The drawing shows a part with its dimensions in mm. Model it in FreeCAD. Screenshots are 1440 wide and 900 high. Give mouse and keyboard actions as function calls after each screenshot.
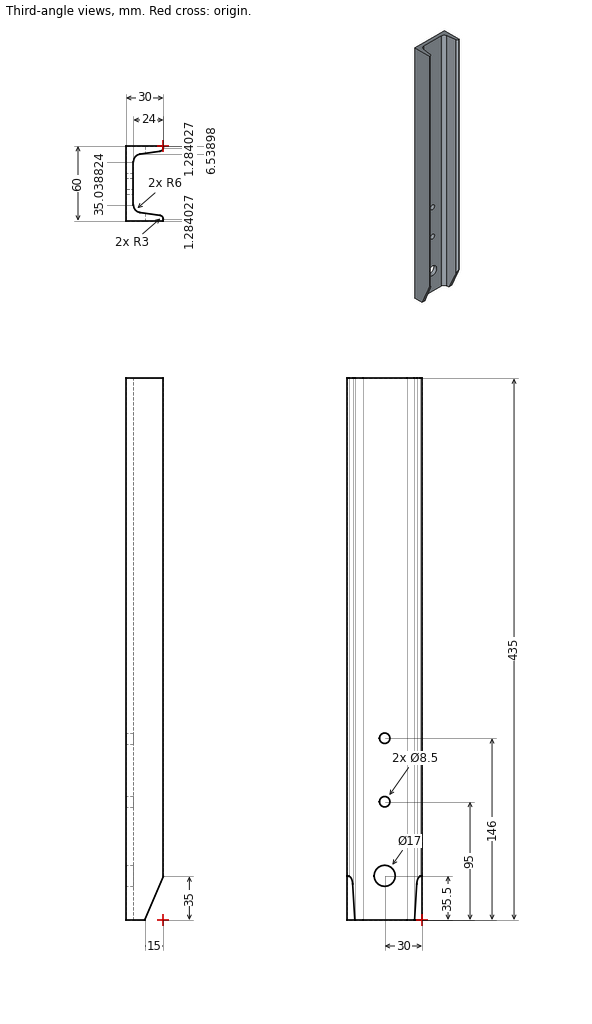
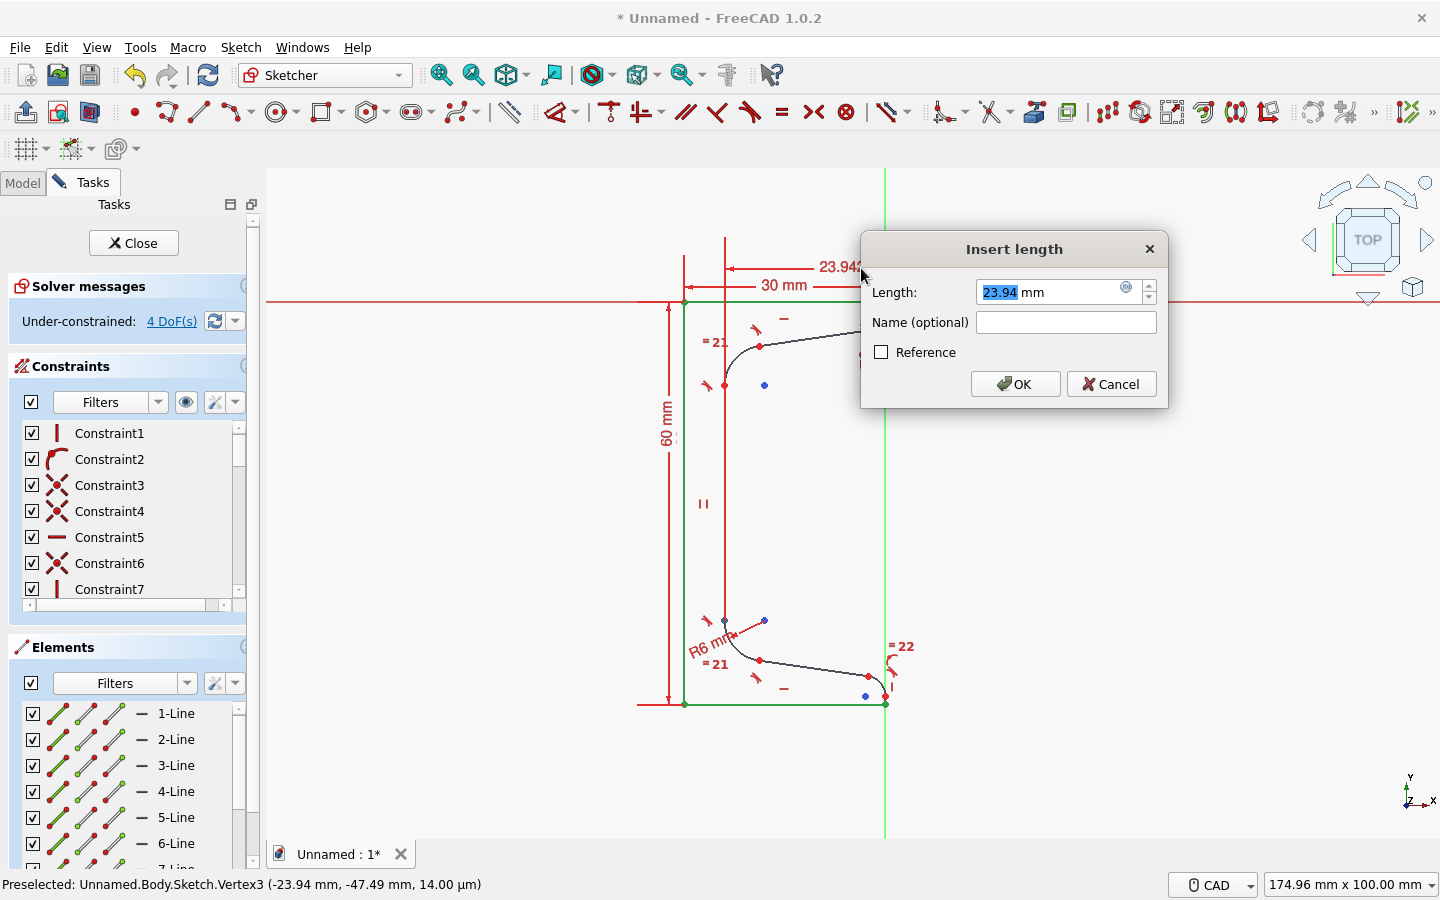
text(24)
key(Return)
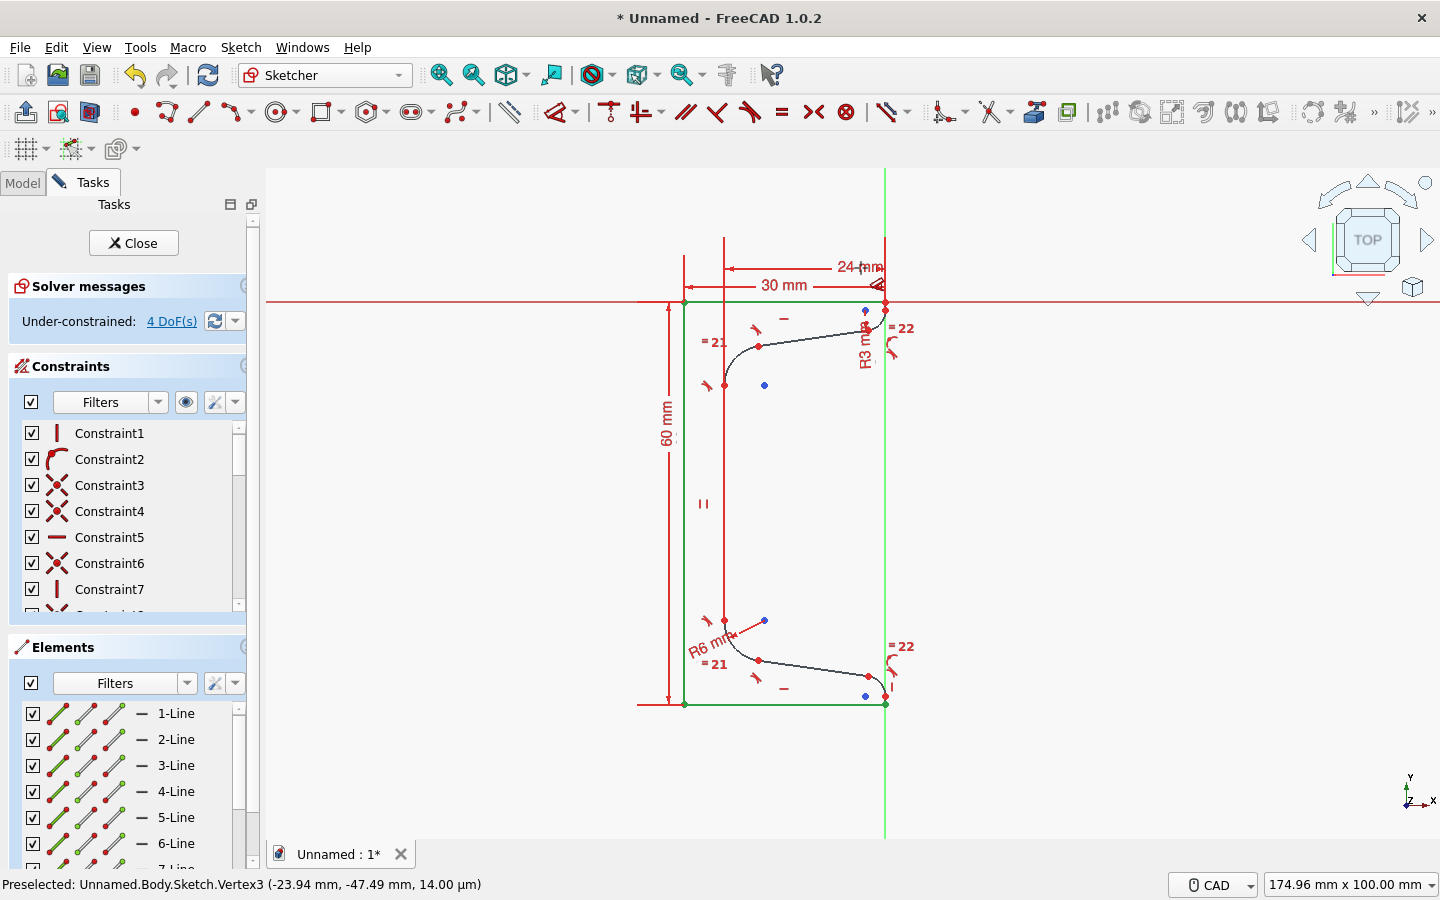
scroll(885, 306, up, 8)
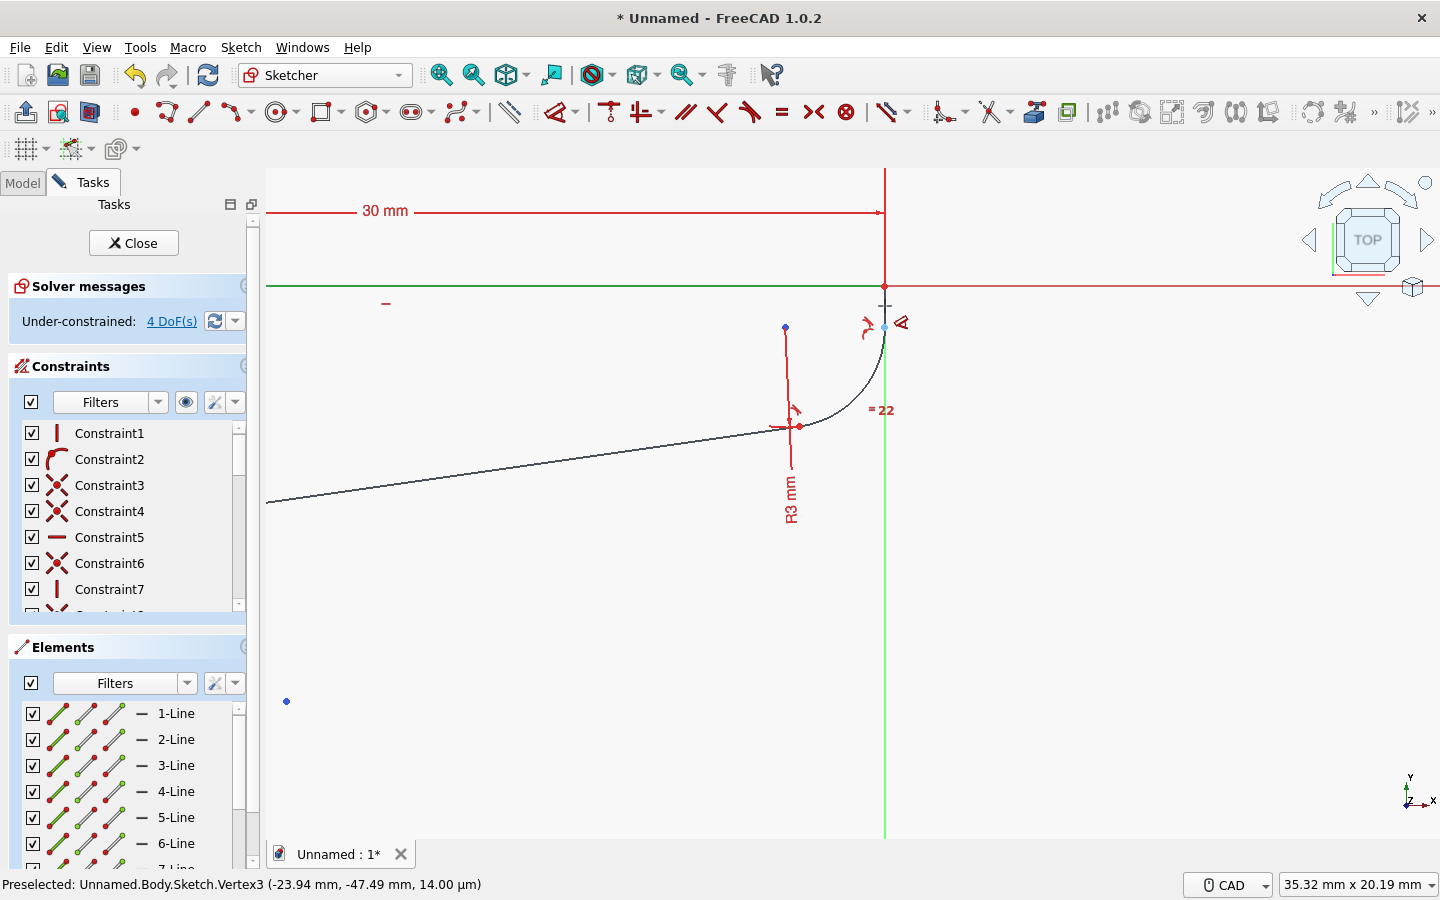
click(885, 307)
click(919, 307)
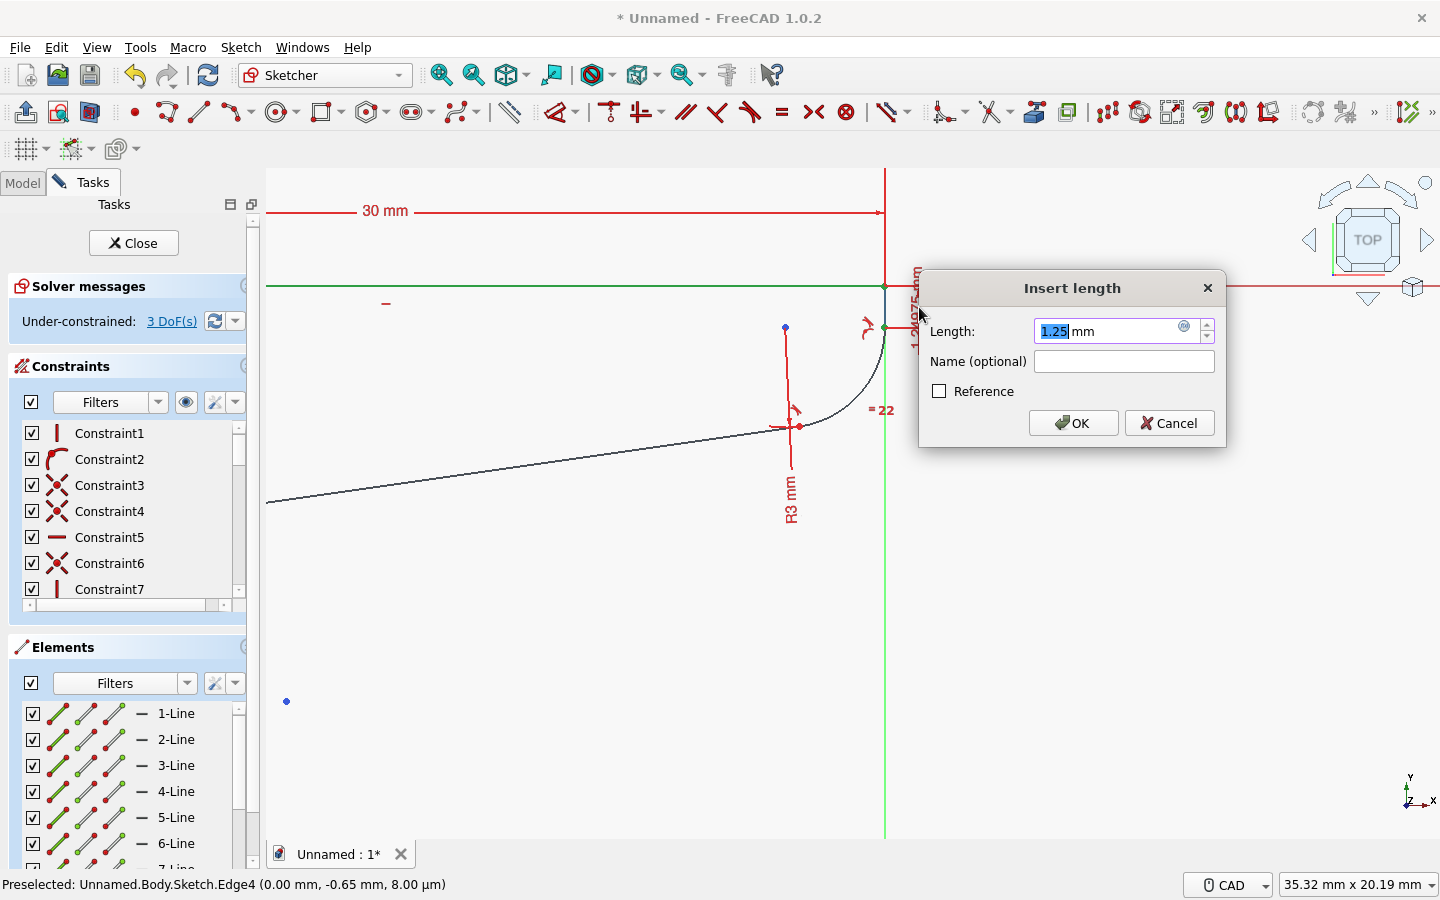
text(1.284027)
key(Return)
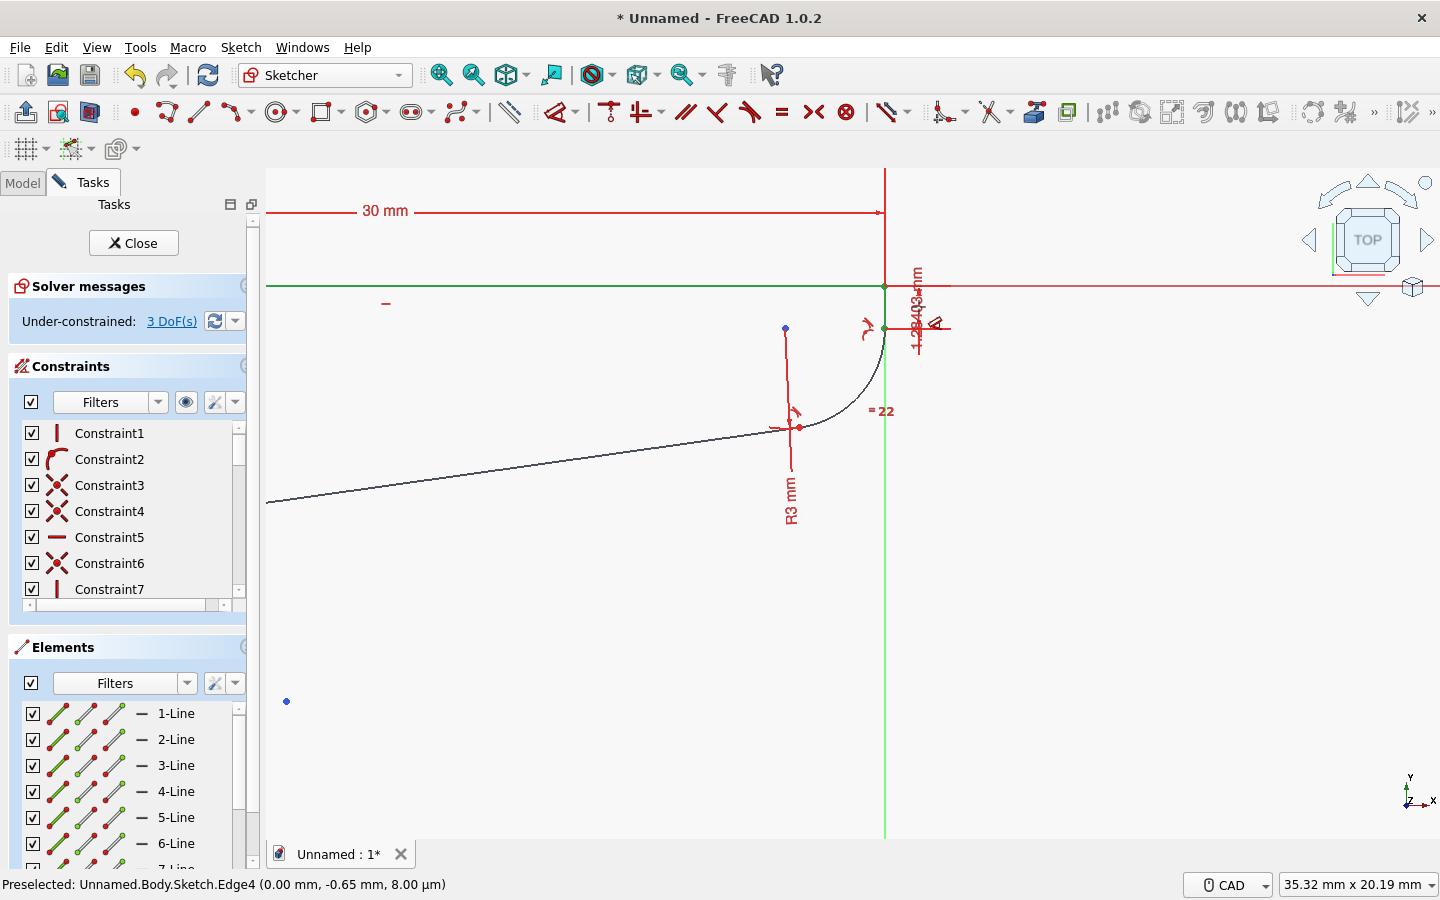
scroll(885, 306, down, 8)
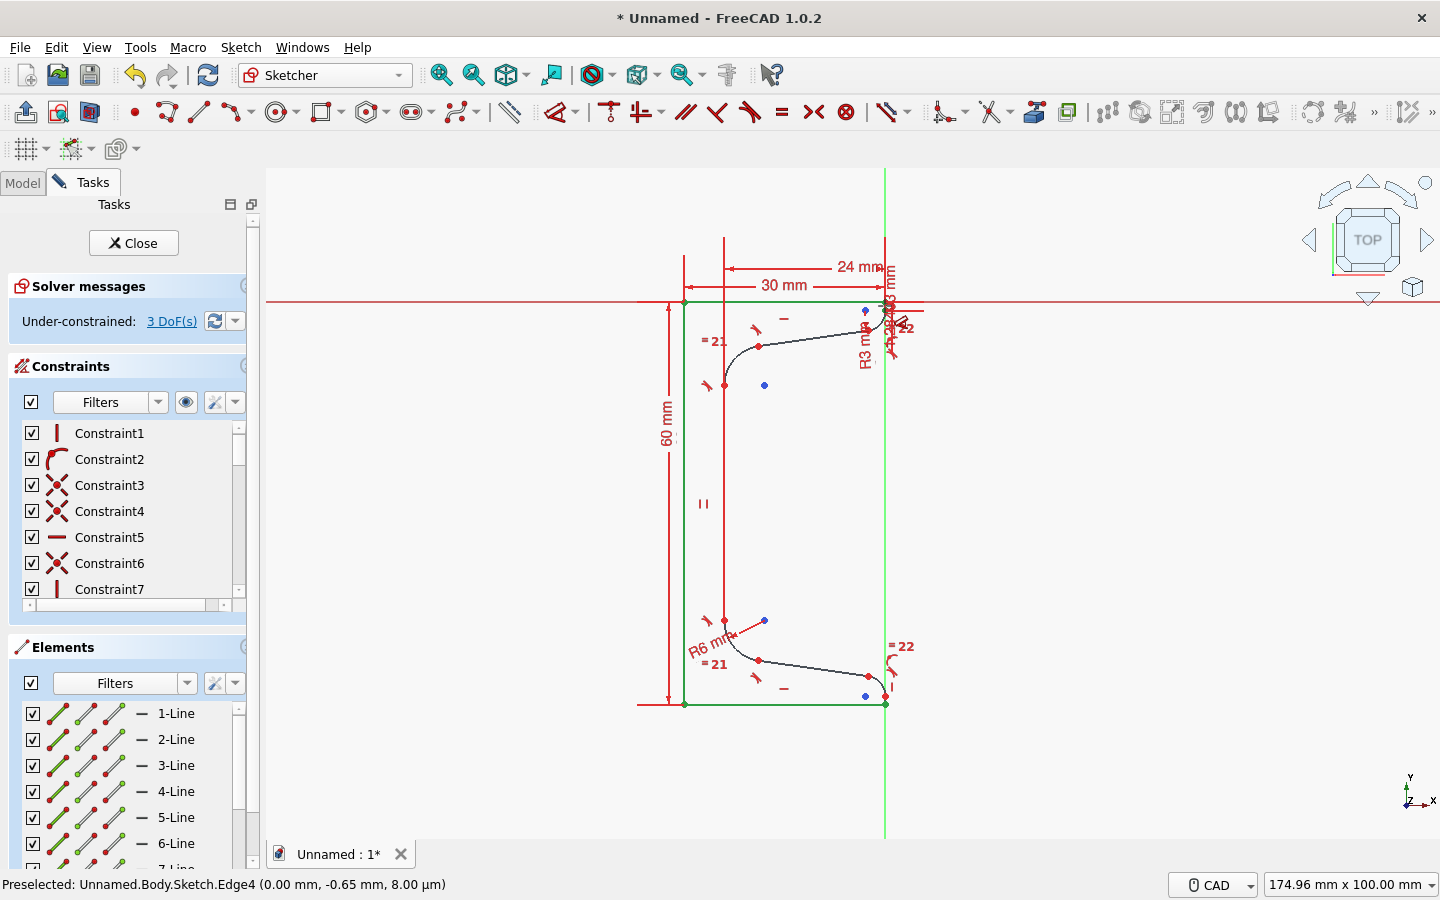
scroll(885, 702, up, 9)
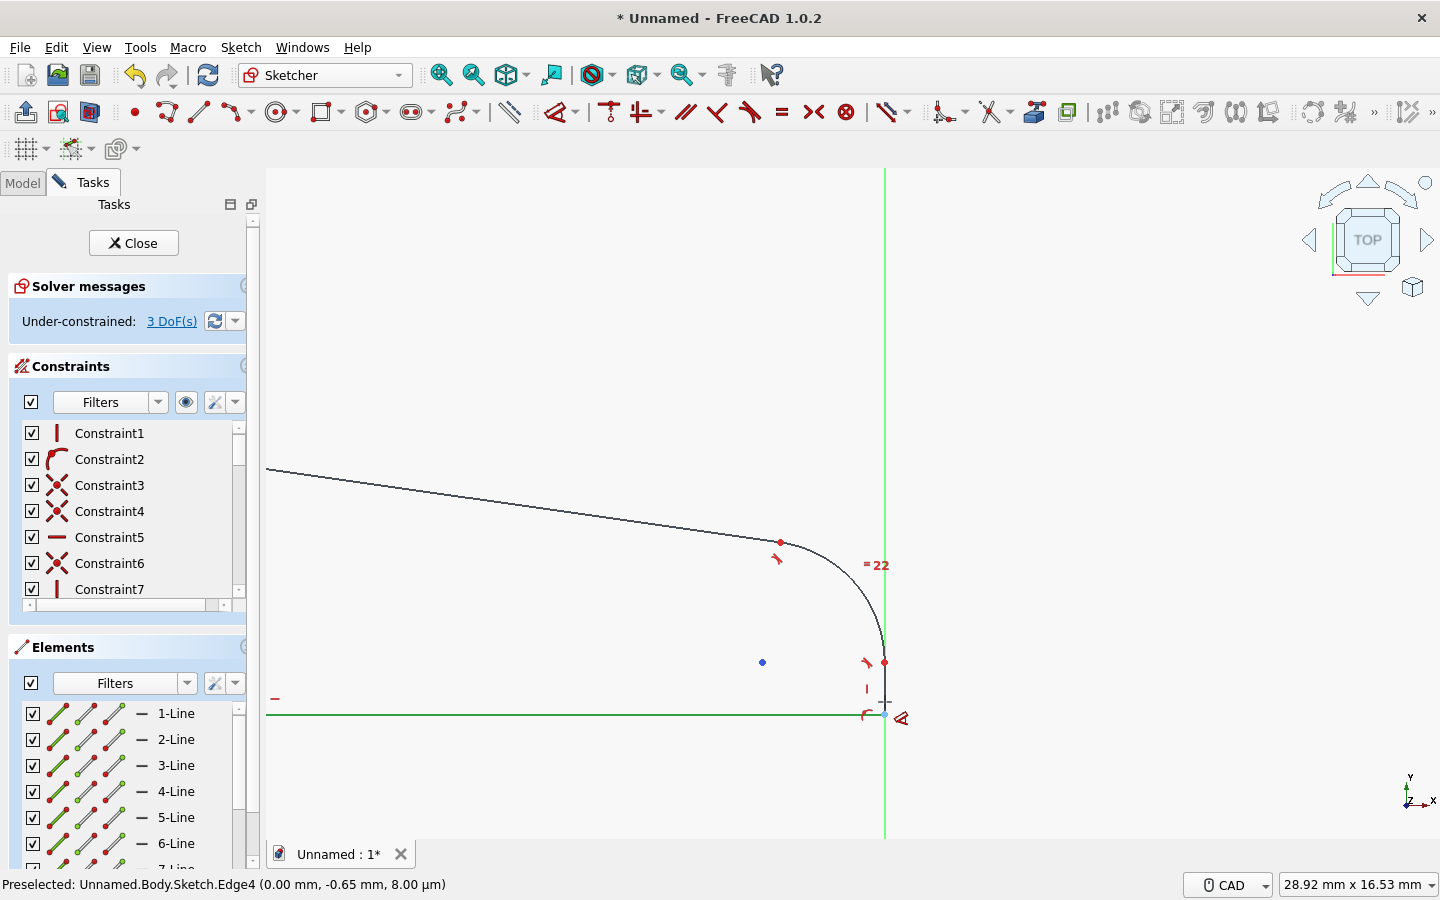
click(885, 699)
click(919, 689)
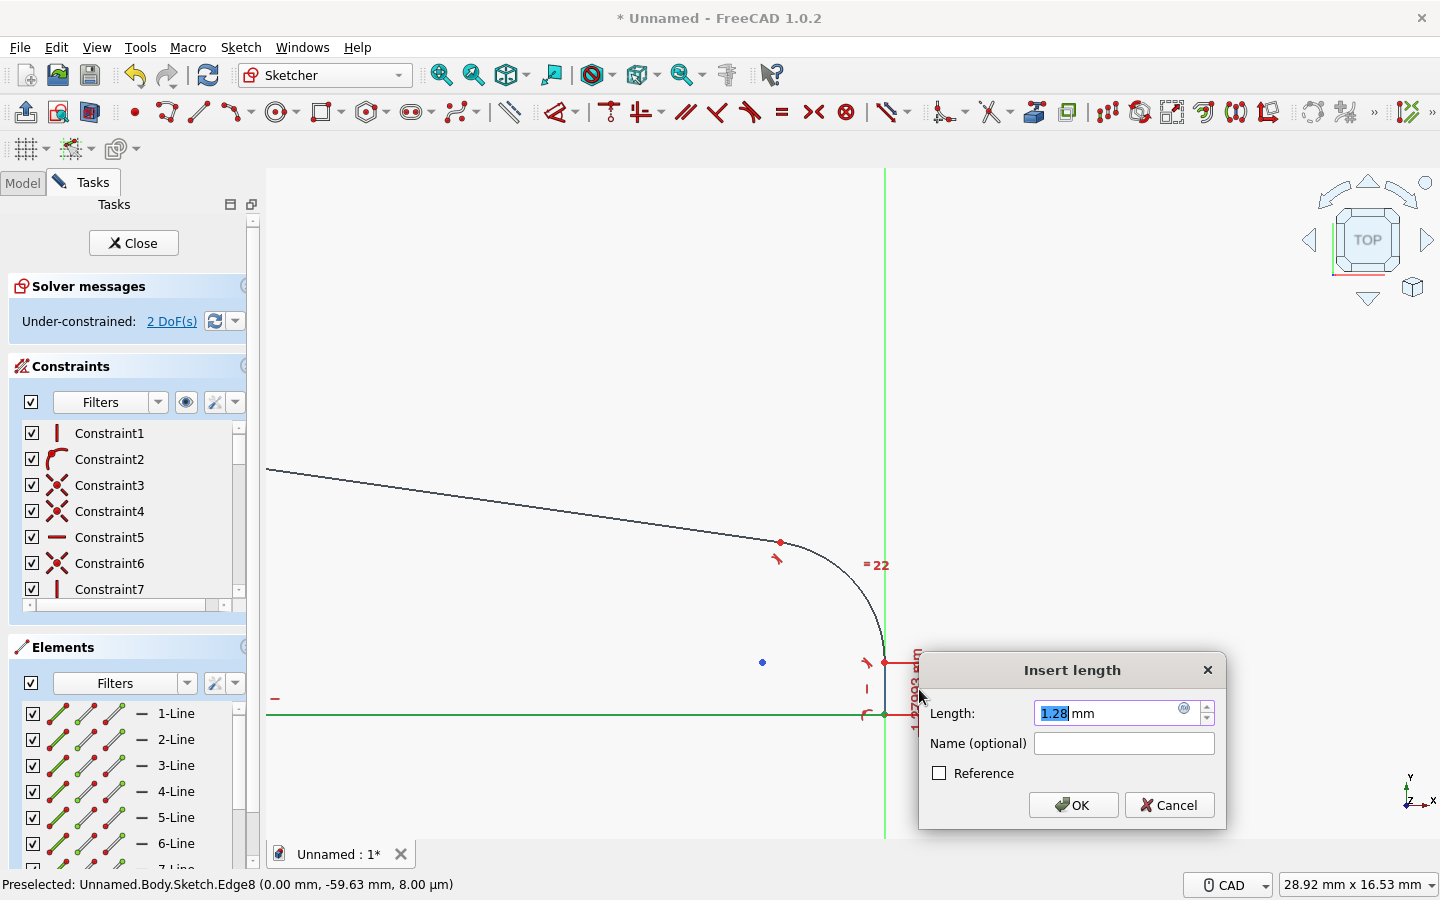
text(1.284027)
key(Return)